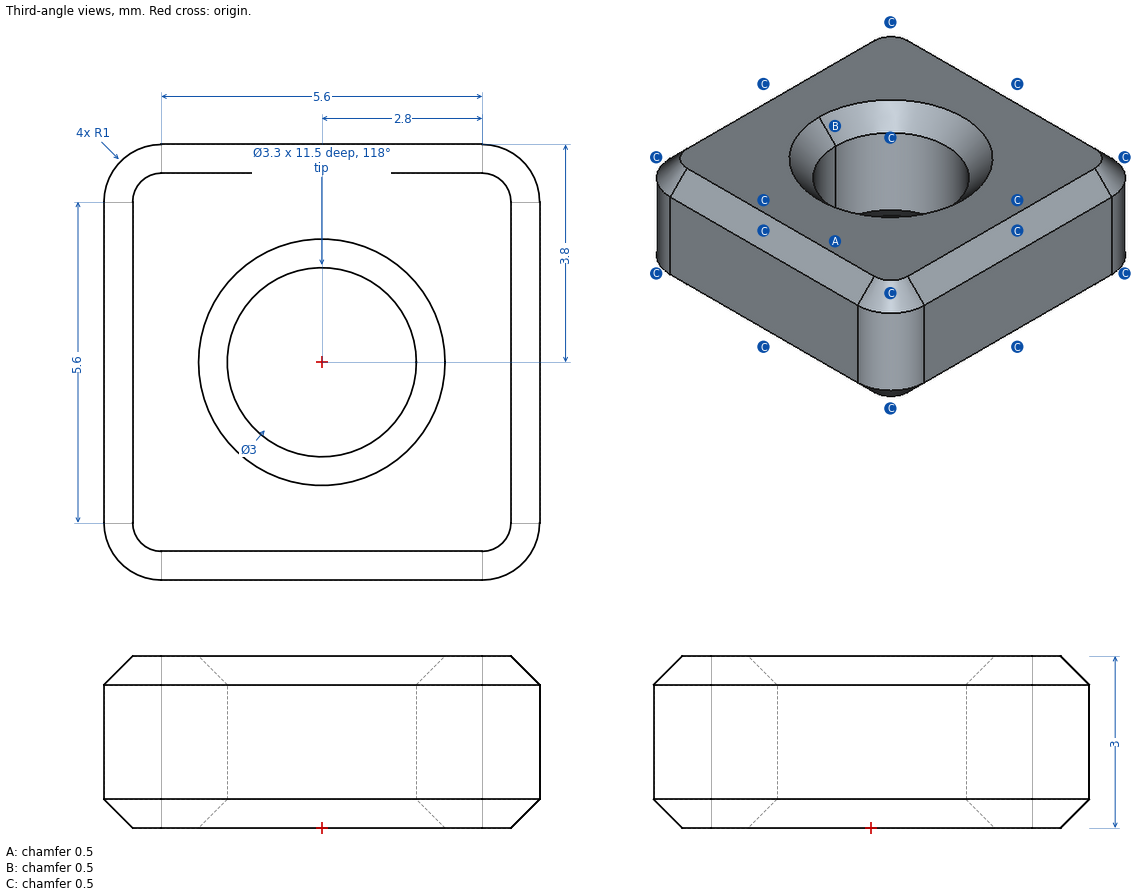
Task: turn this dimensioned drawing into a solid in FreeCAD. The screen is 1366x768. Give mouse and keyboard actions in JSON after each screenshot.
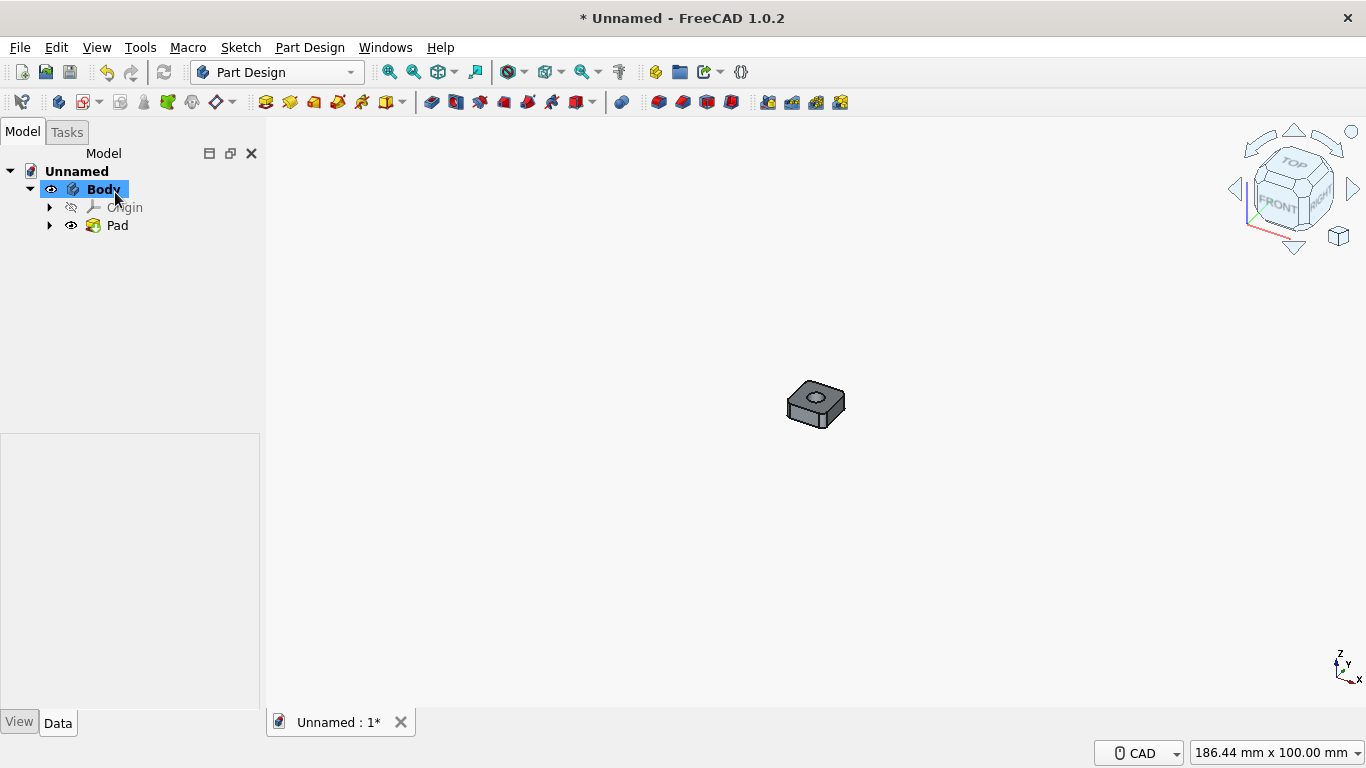
{"action": "key", "text": "v f"}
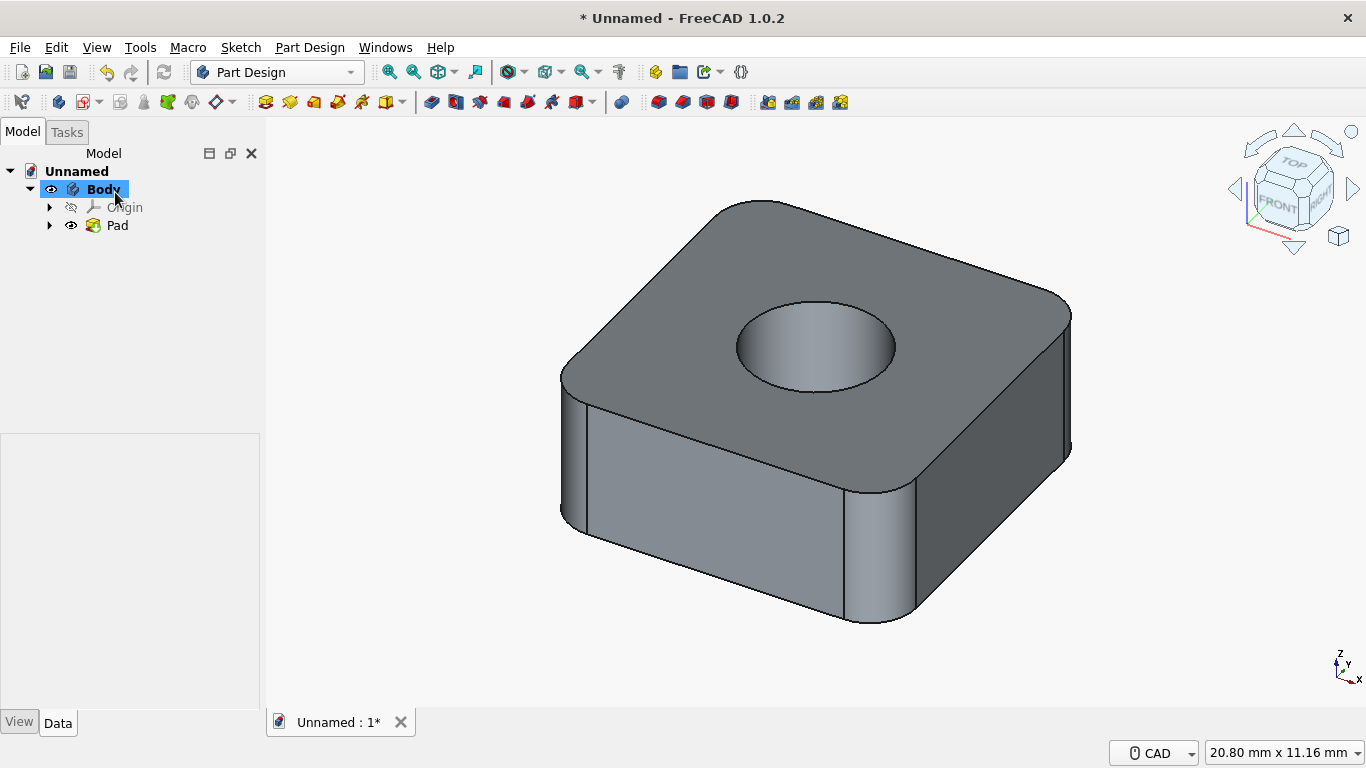
{"action": "key", "text": "5"}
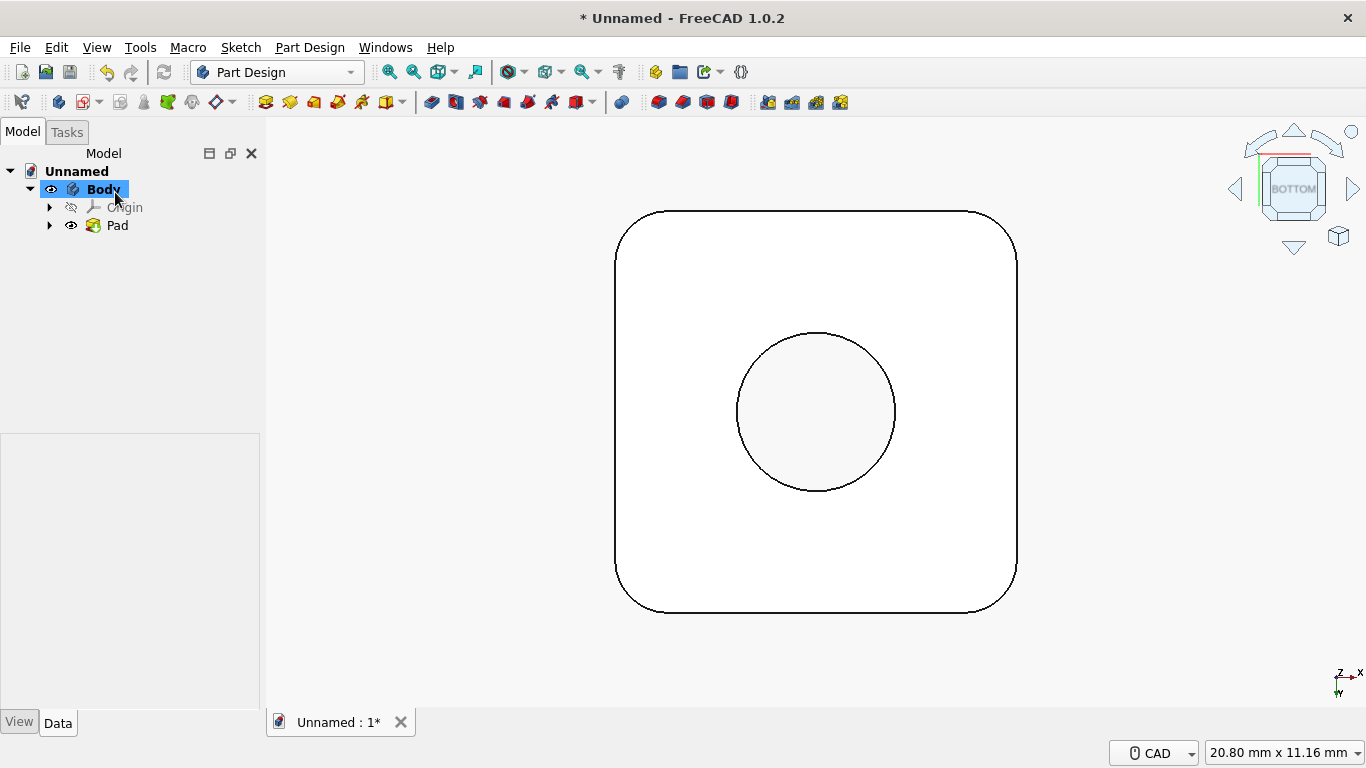
{"action": "left_click", "coordinate": [701, 296]}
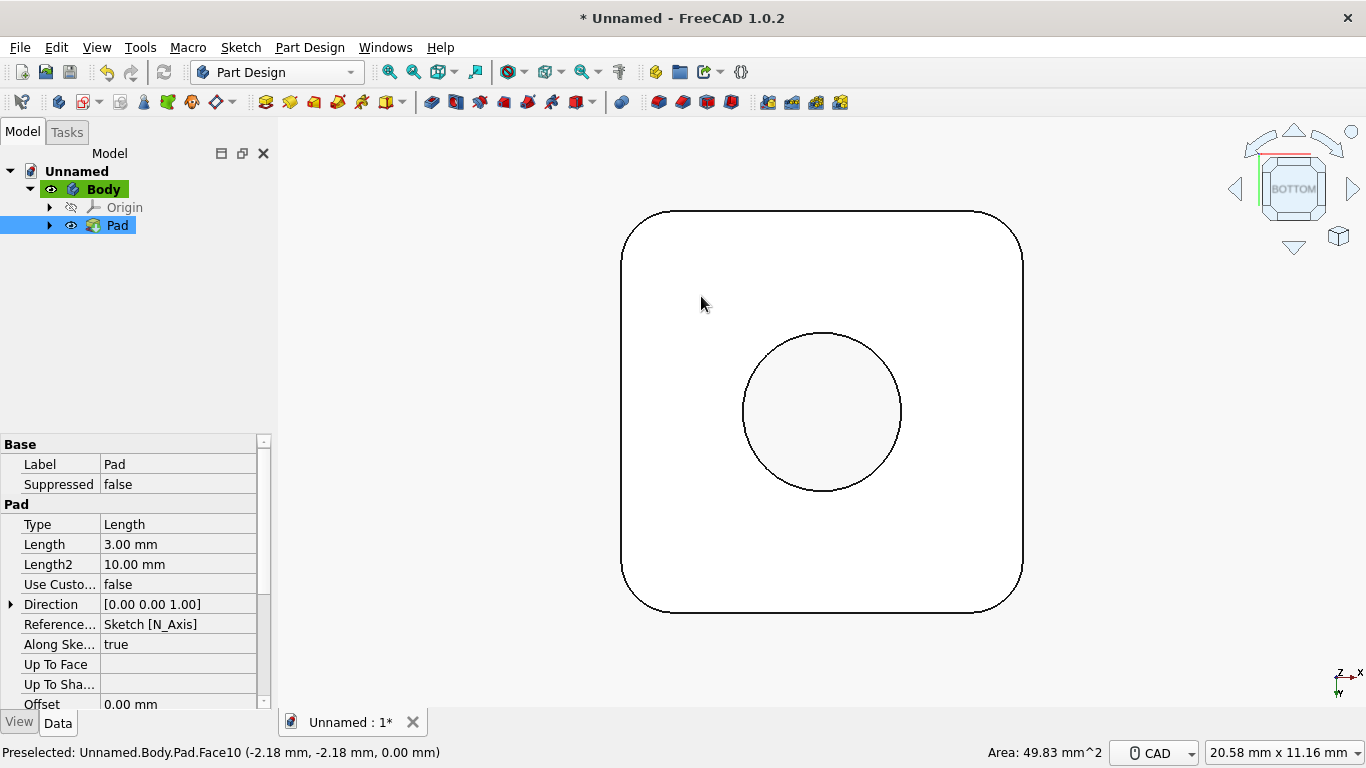
{"action": "left_click", "coordinate": [84, 102]}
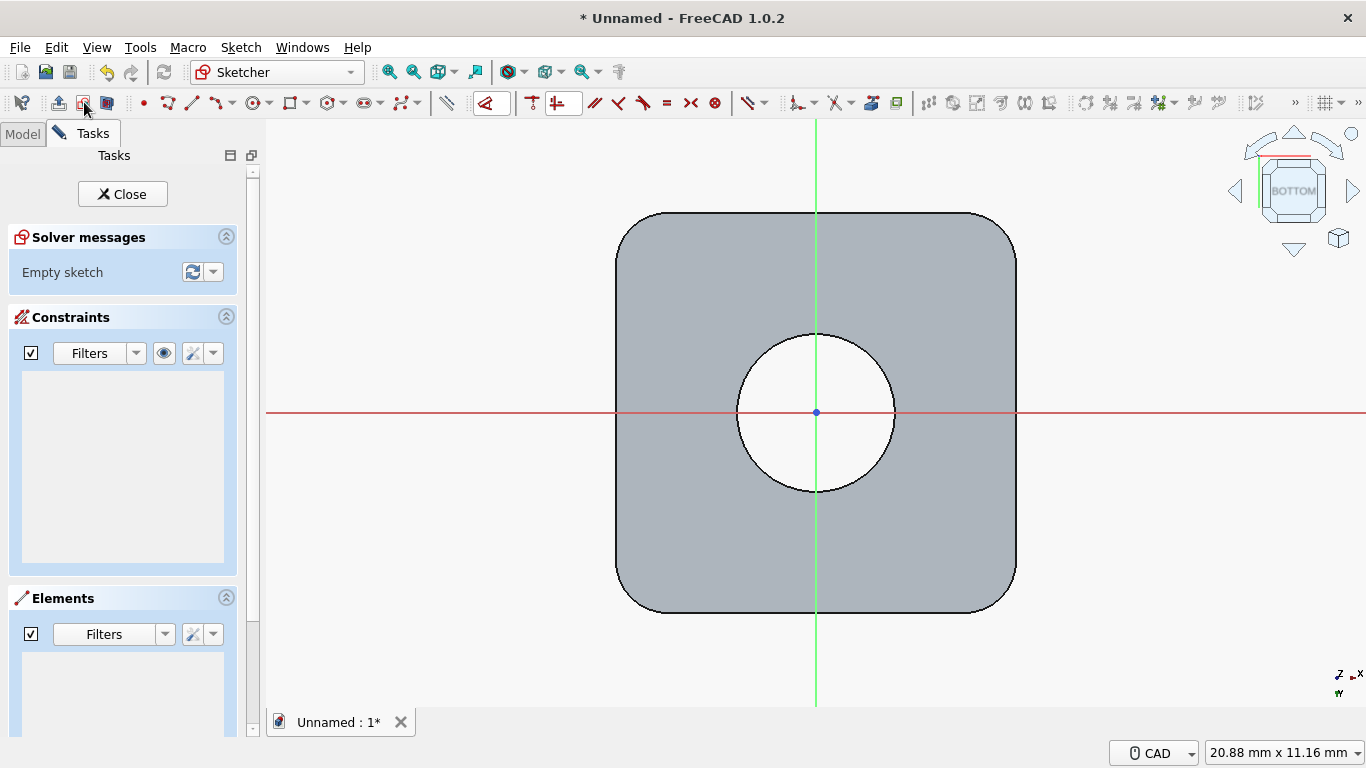
{"action": "scroll", "coordinate": [872, 413], "scroll_direction": "up", "scroll_amount": 4}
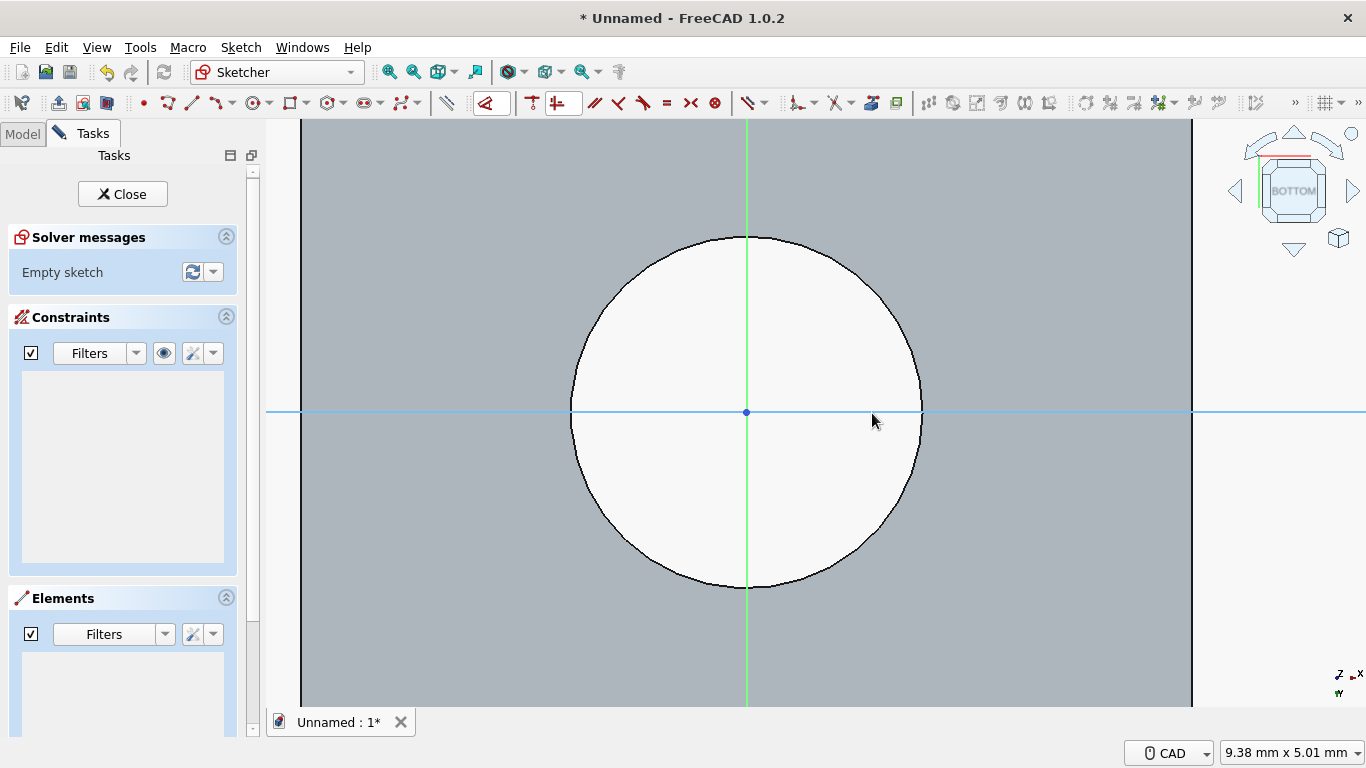
{"action": "key", "text": "g c"}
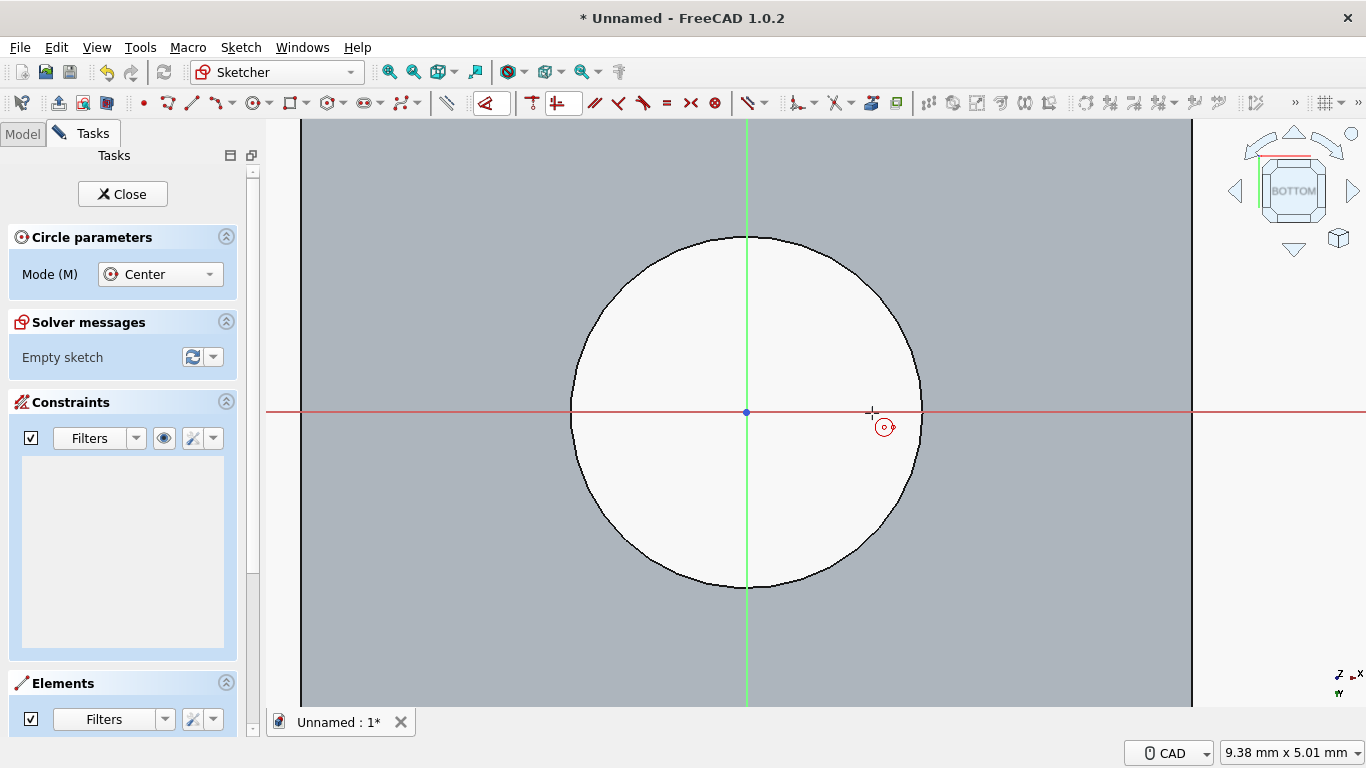
{"action": "left_click", "coordinate": [747, 412]}
{"action": "left_click", "coordinate": [884, 276]}
{"action": "key", "text": "Escape"}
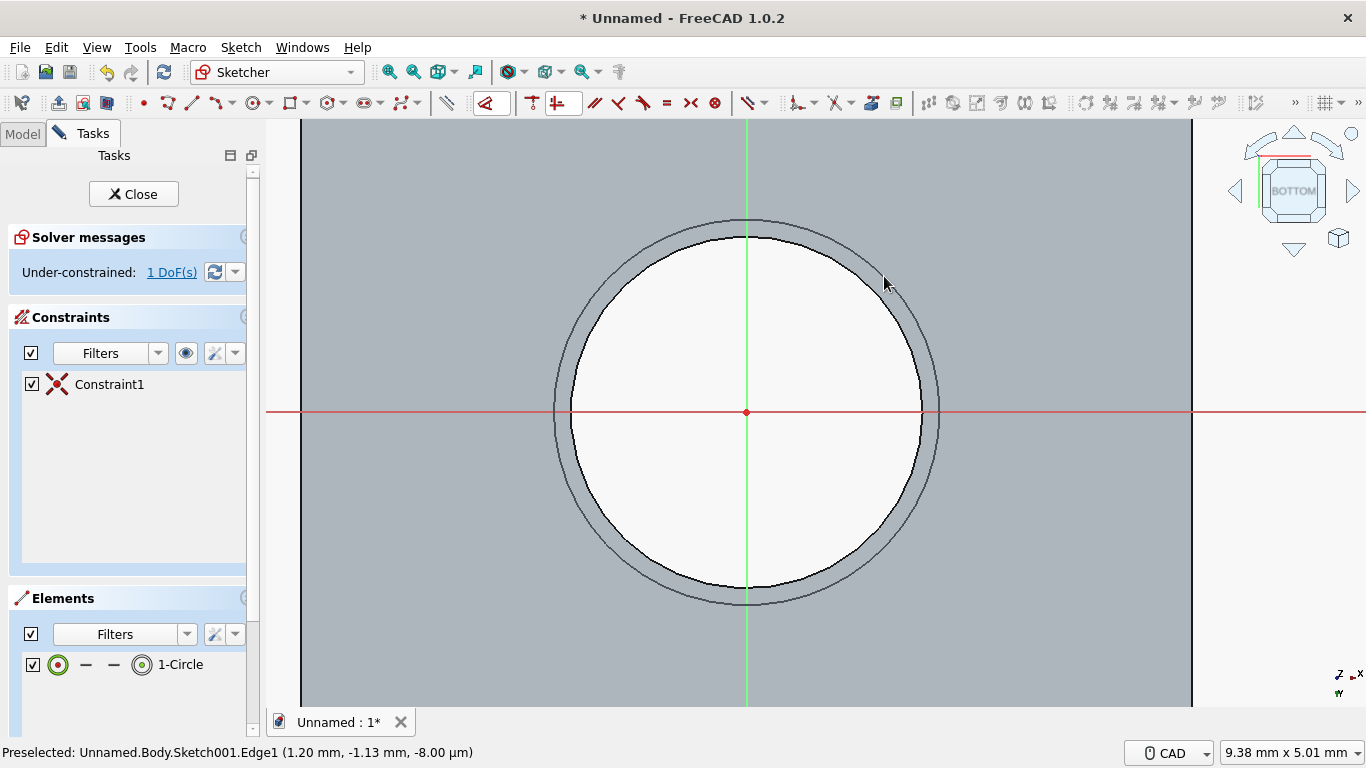
{"action": "key", "text": "d"}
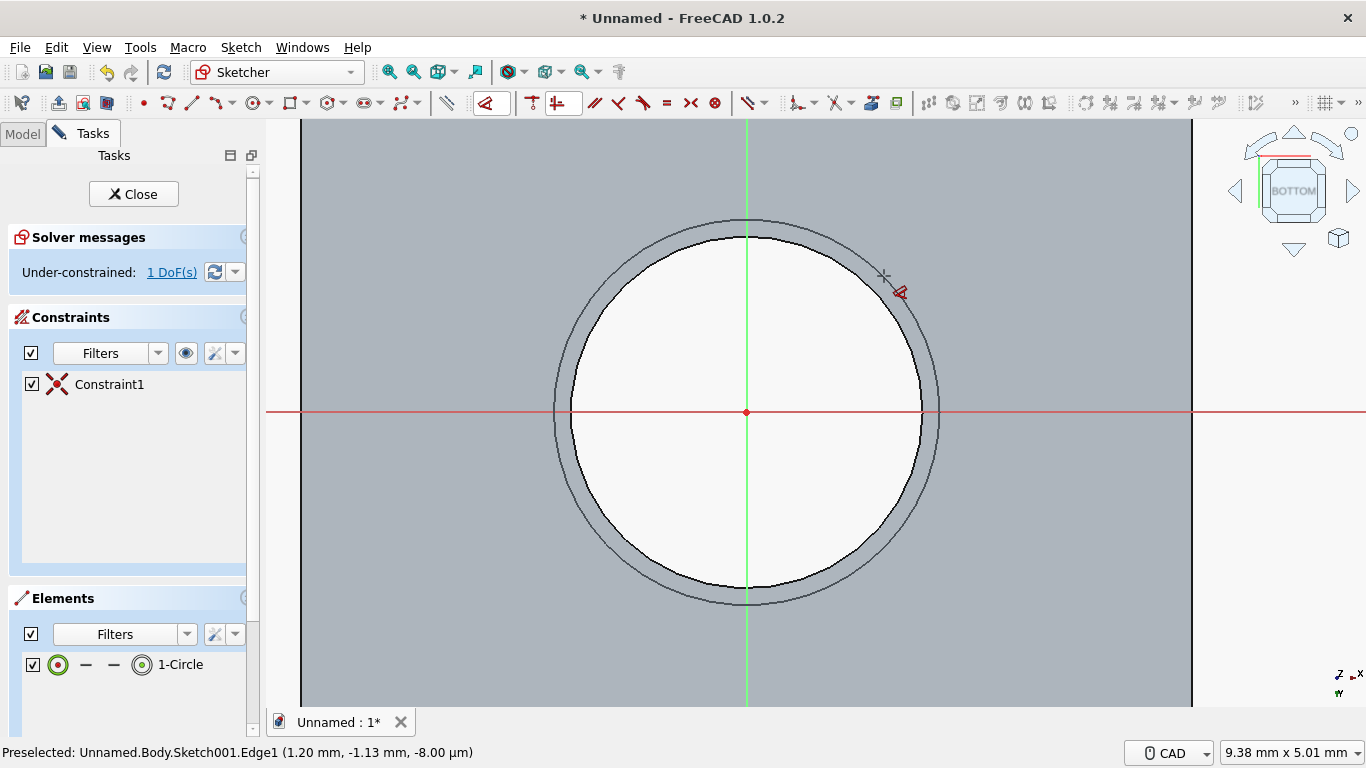
{"action": "left_click", "coordinate": [883, 276]}
{"action": "left_click", "coordinate": [906, 253]}